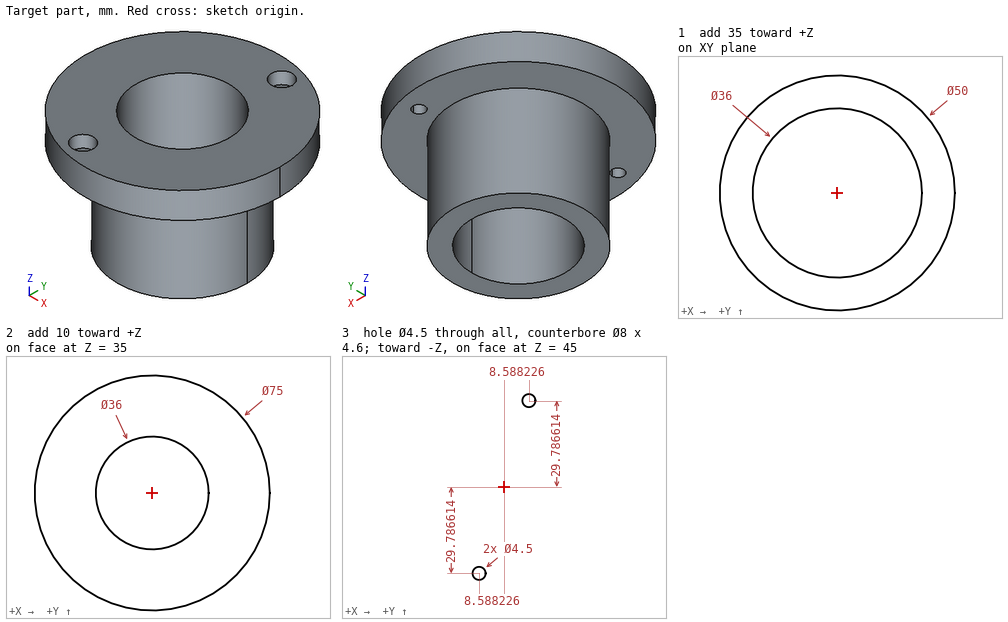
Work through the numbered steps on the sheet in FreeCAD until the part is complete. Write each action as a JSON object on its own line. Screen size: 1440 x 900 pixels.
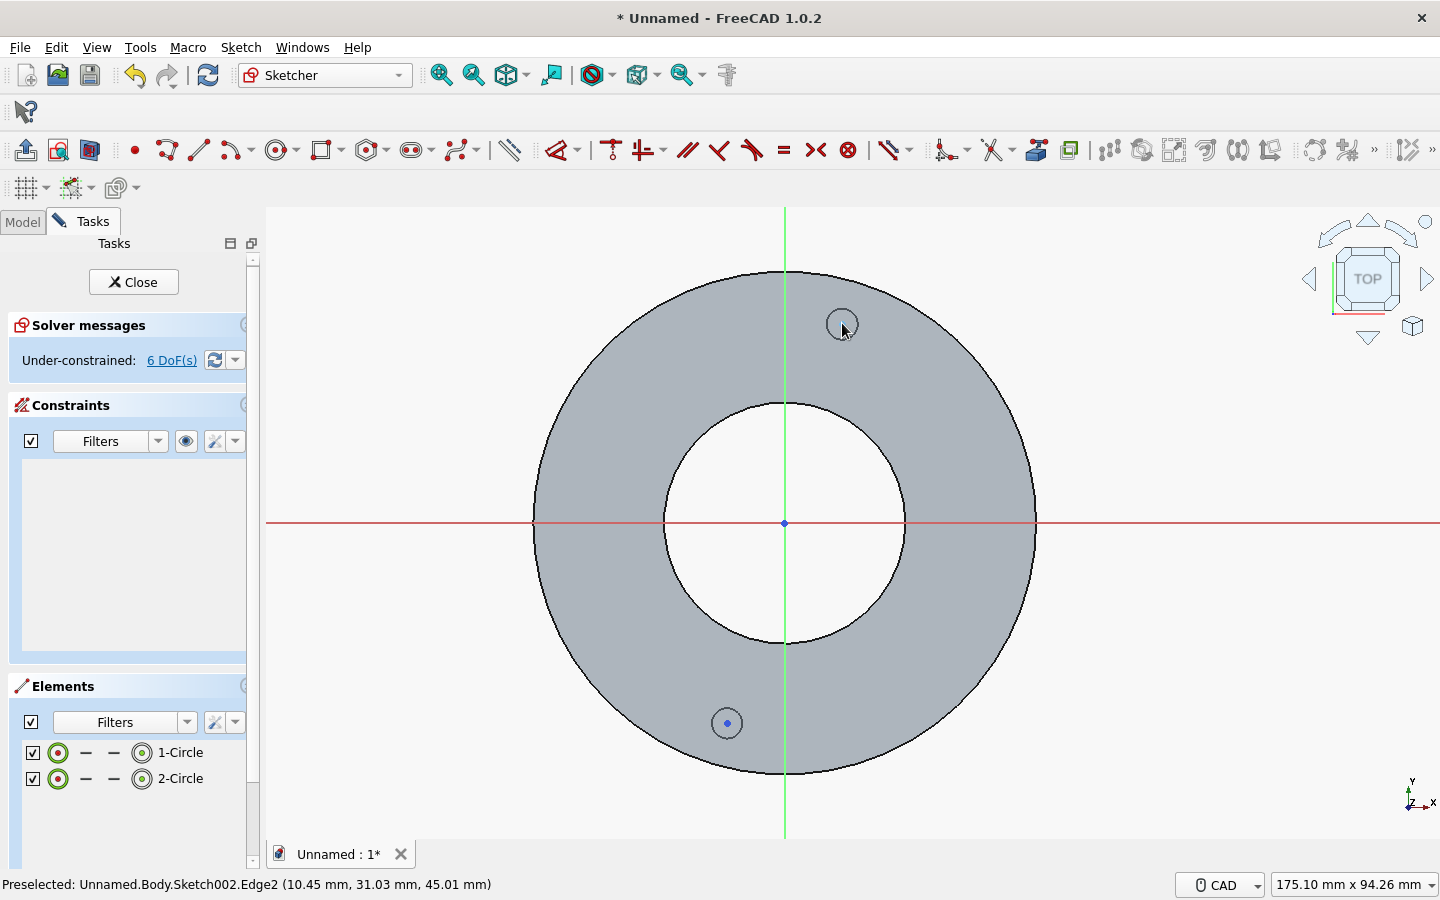
{"action": "left_click", "coordinate": [738, 713]}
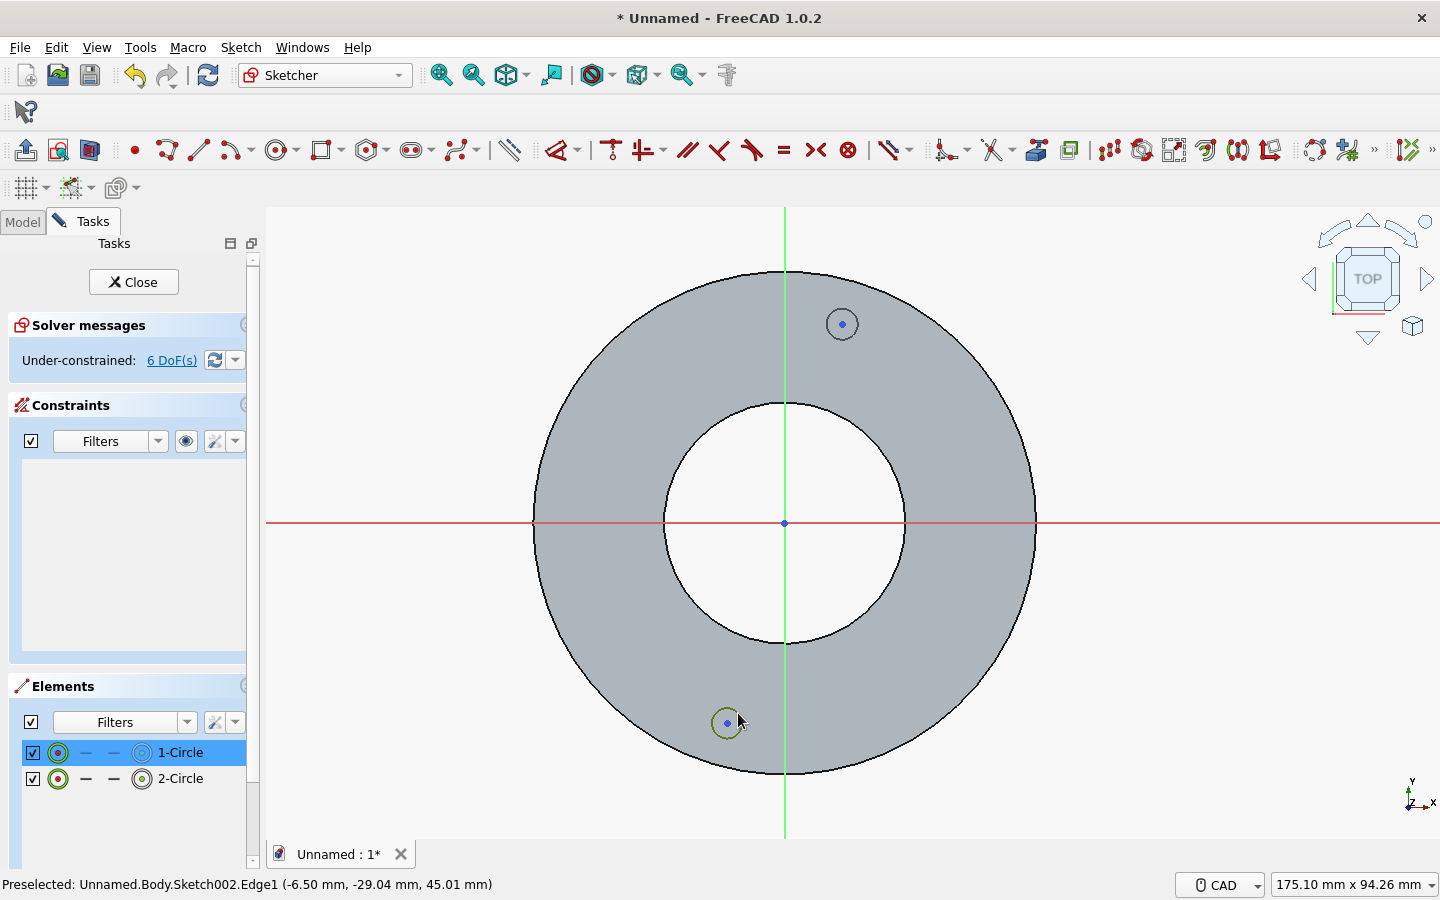
{"action": "left_click", "coordinate": [853, 313]}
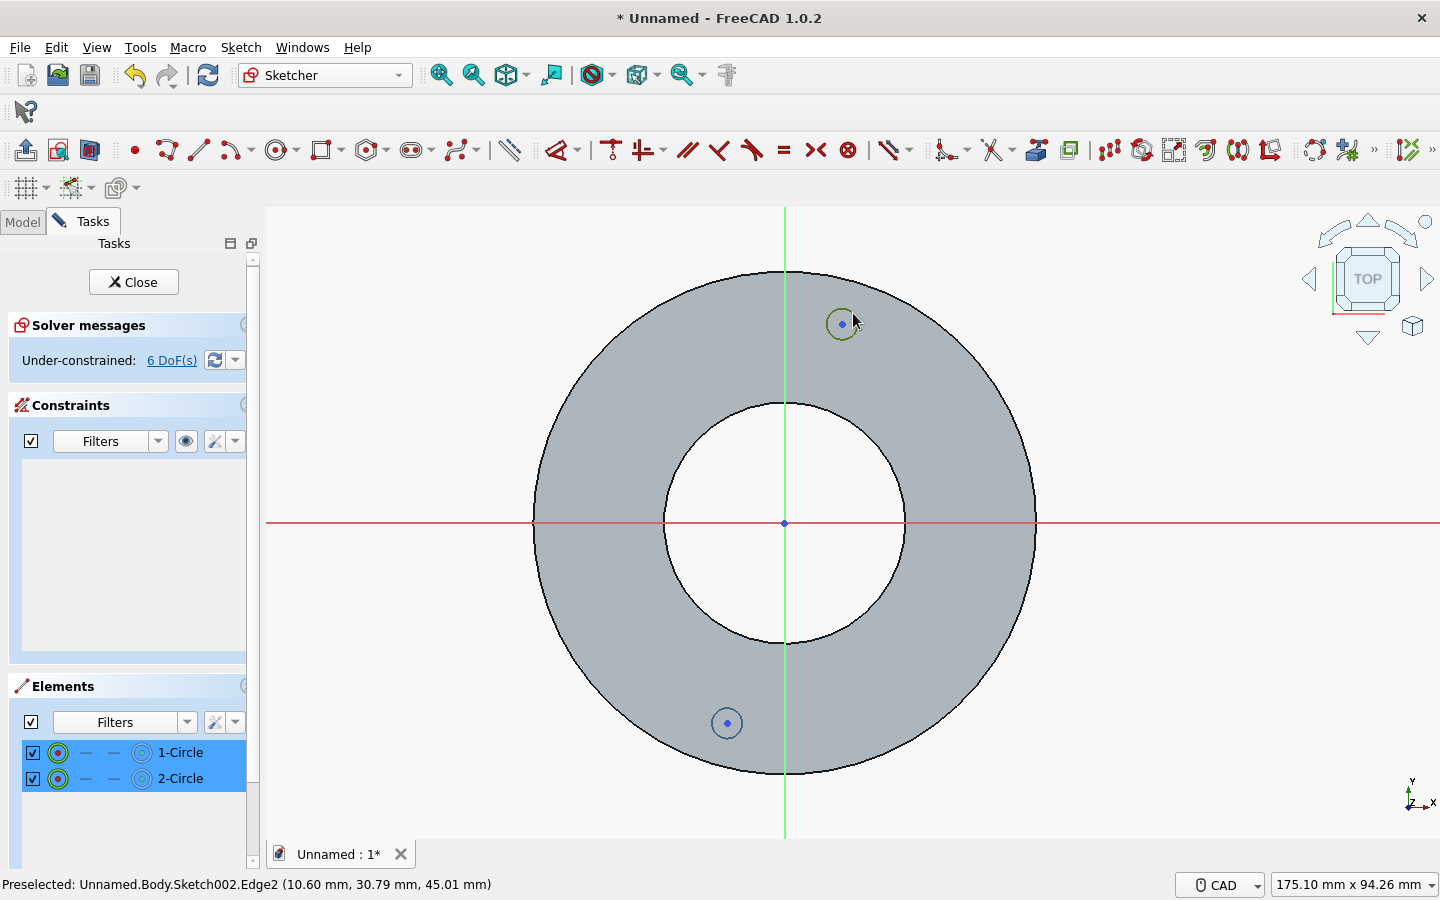
{"action": "left_click", "coordinate": [784, 150]}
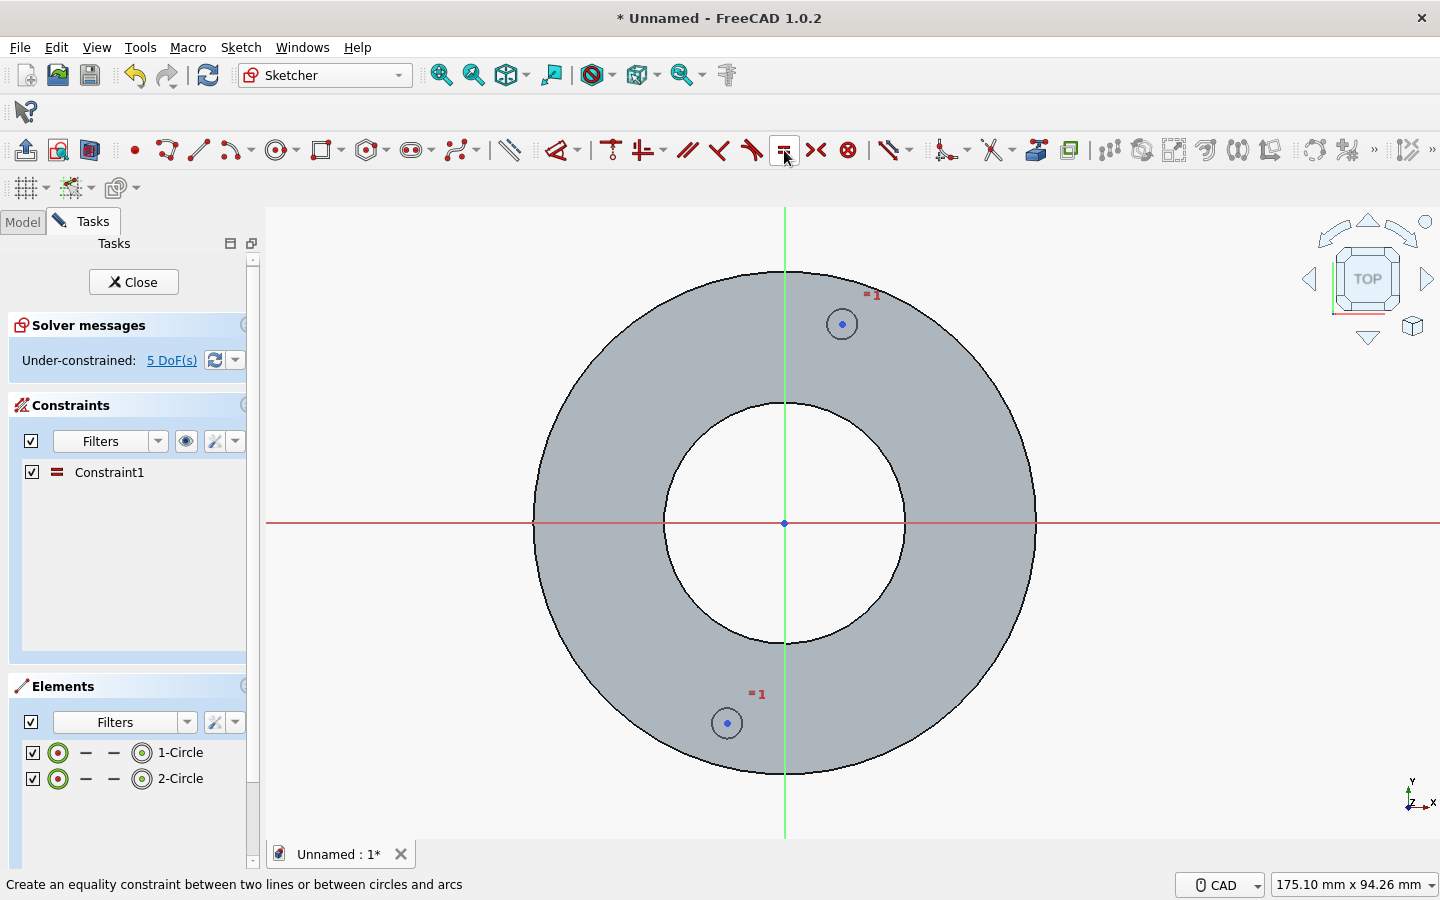
{"action": "key", "text": "d"}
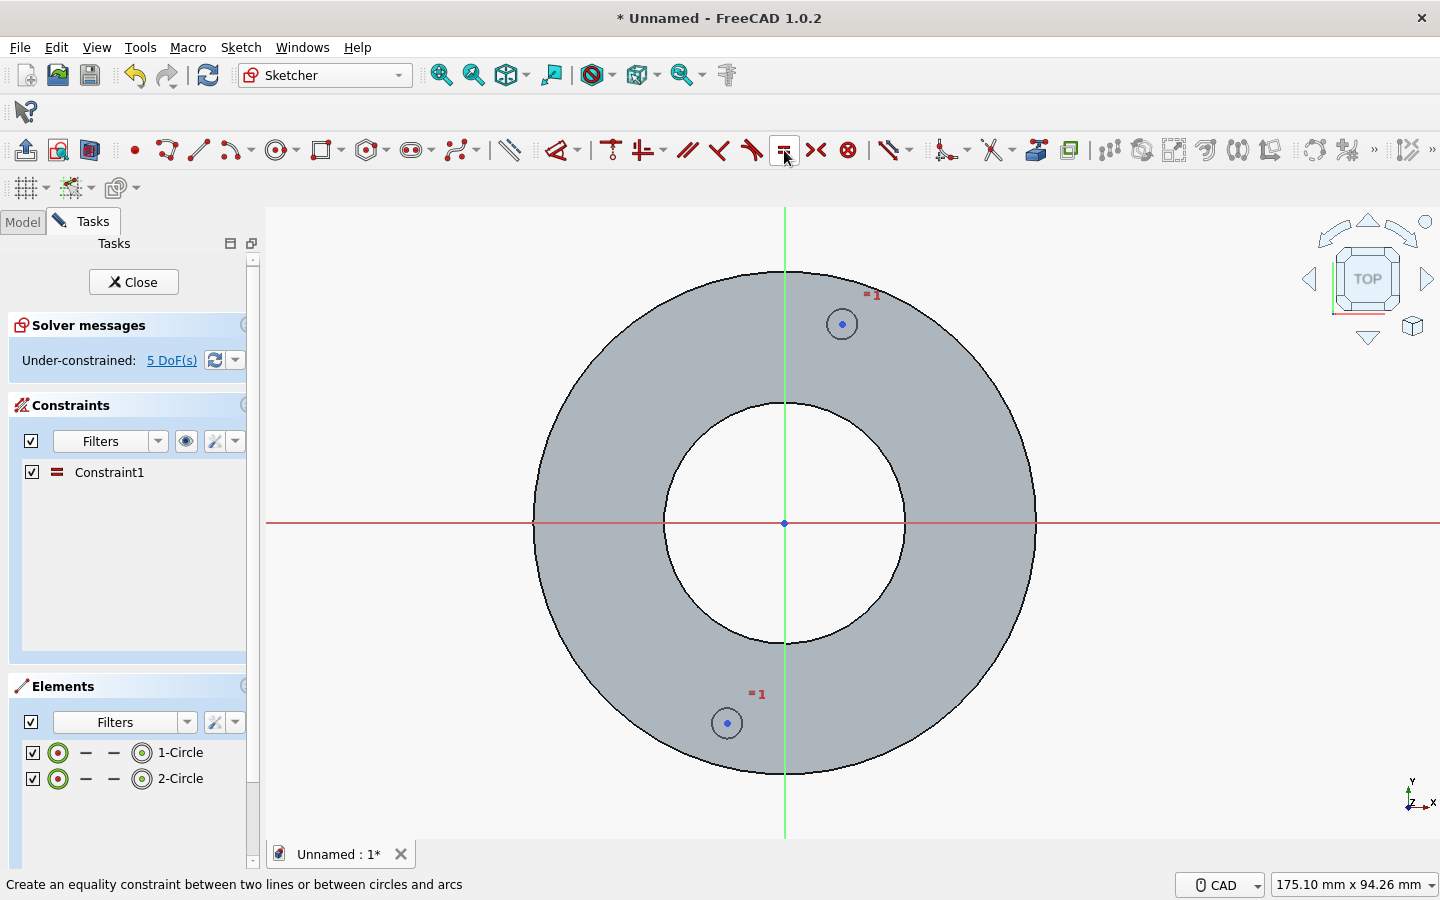
{"action": "scroll", "coordinate": [738, 713], "scroll_direction": "up", "scroll_amount": 2}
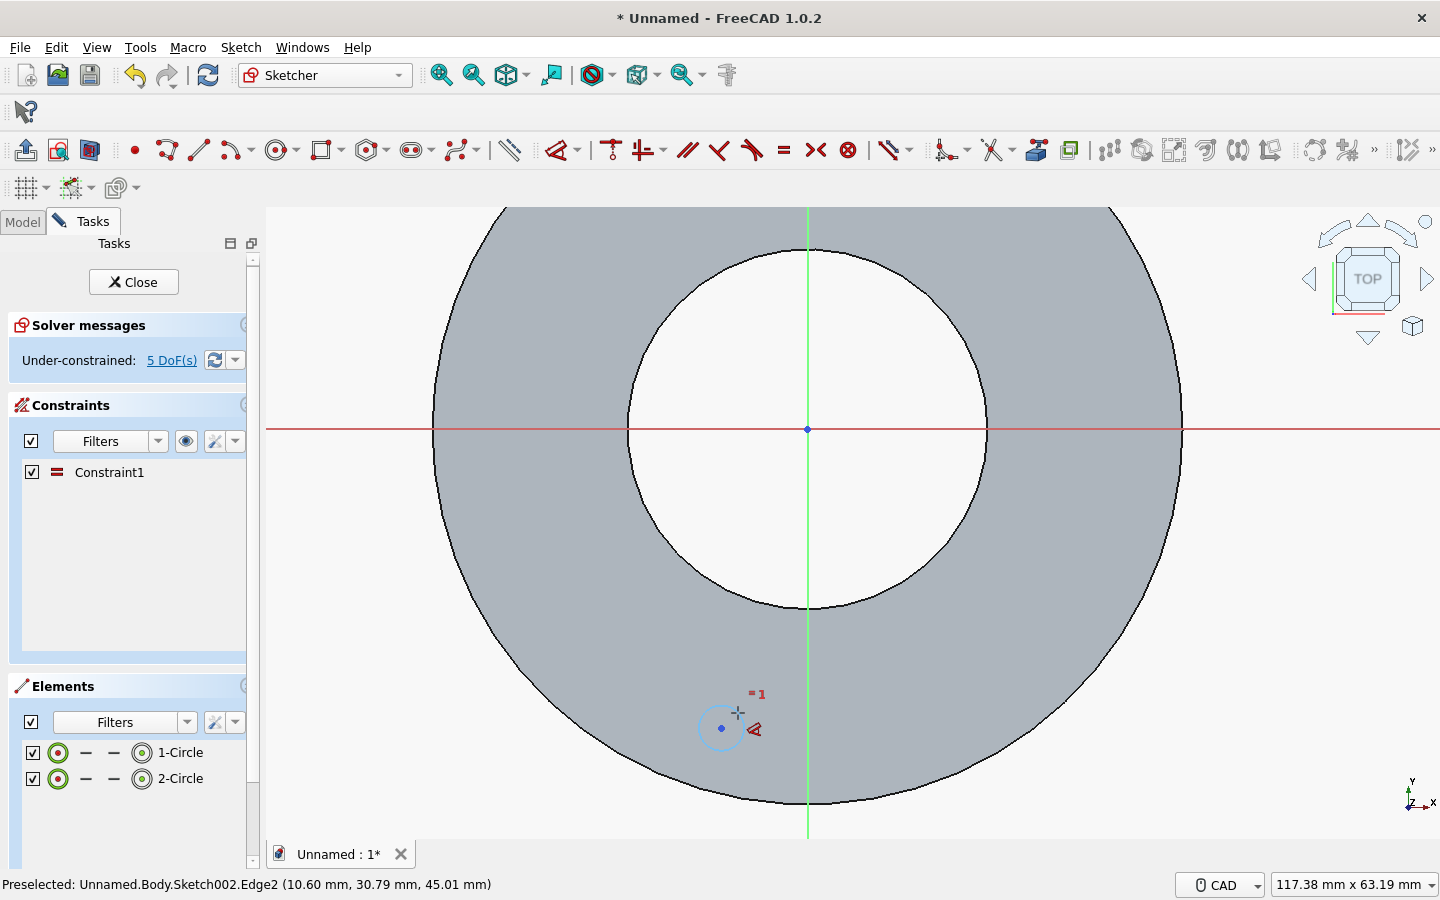
{"action": "left_click", "coordinate": [737, 712]}
{"action": "left_click", "coordinate": [759, 689]}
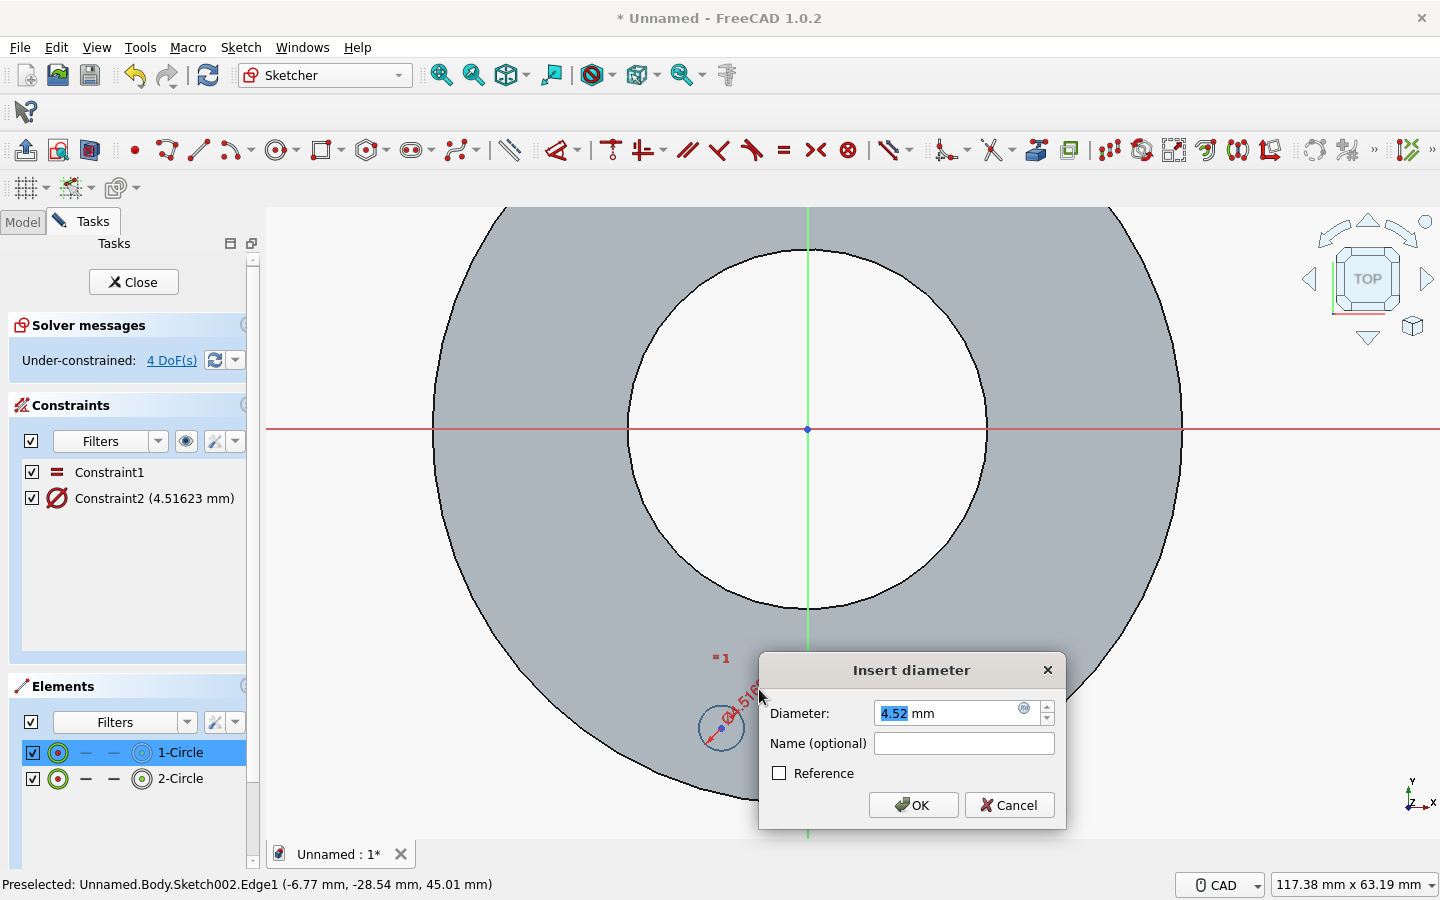
{"action": "type", "text": "4.5"}
{"action": "key", "text": "Return"}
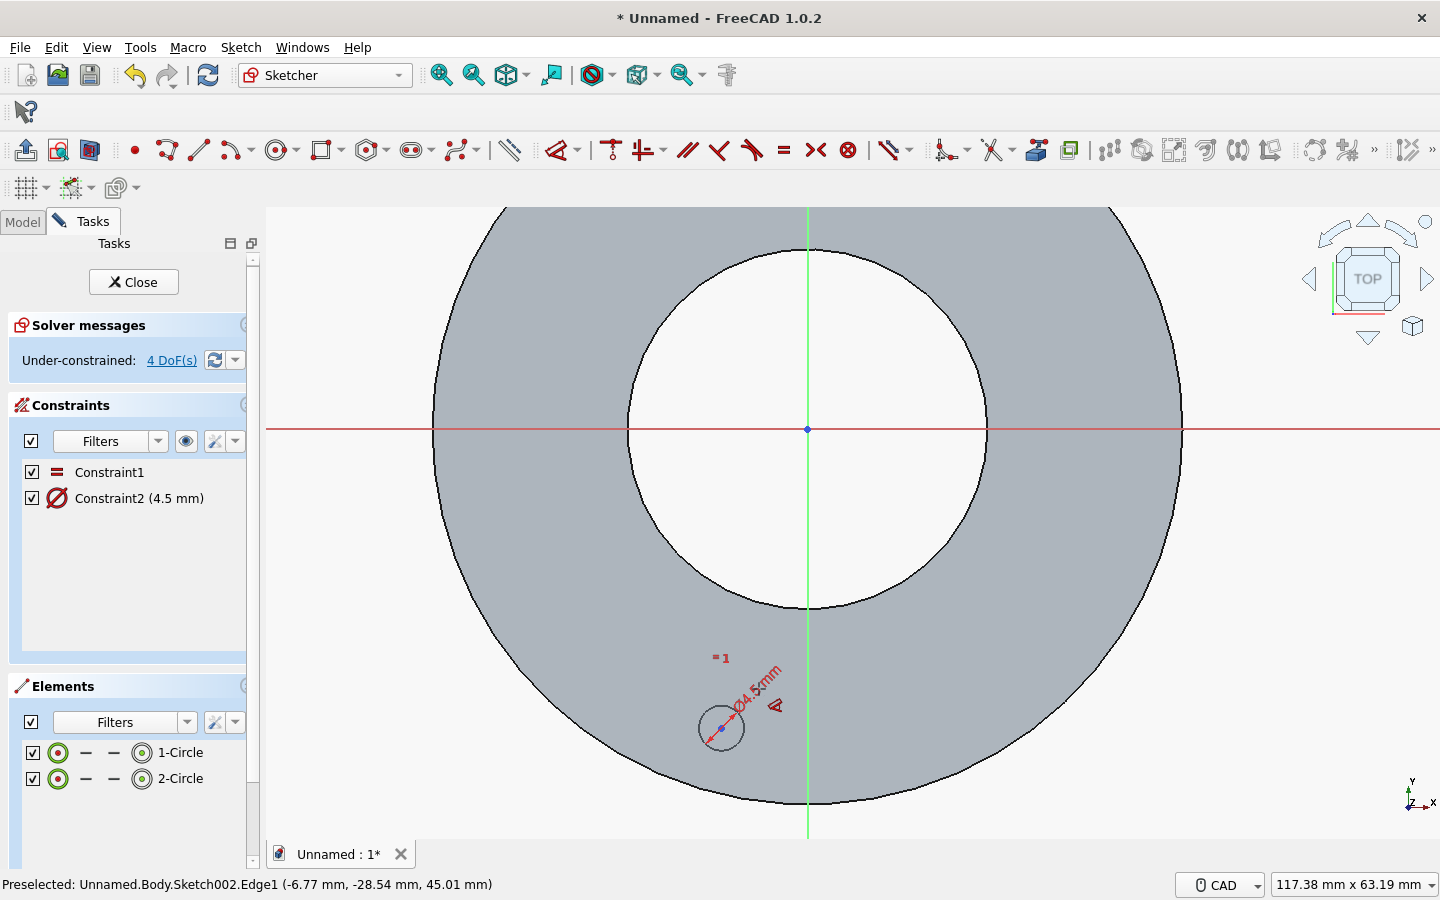
{"action": "left_click", "coordinate": [722, 728]}
{"action": "left_click", "coordinate": [765, 762]}